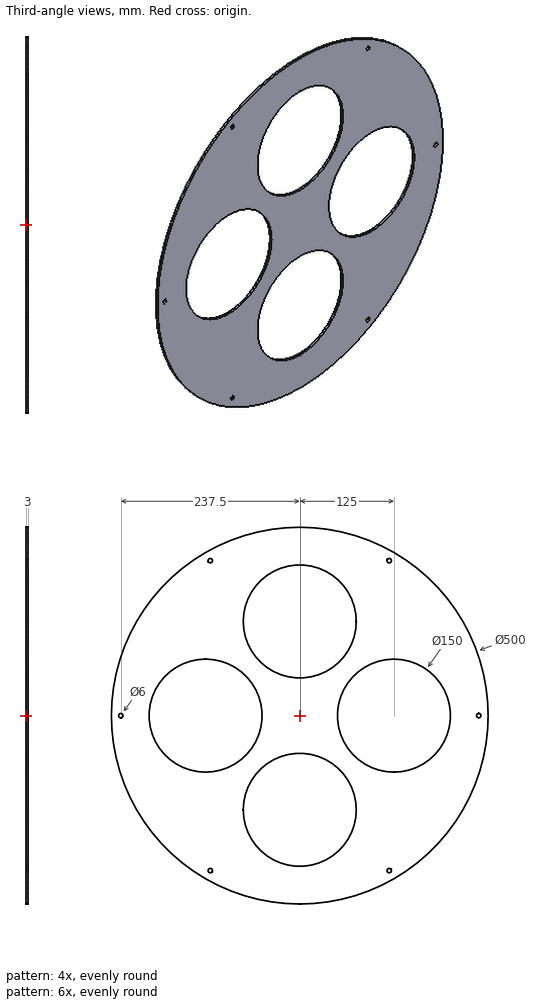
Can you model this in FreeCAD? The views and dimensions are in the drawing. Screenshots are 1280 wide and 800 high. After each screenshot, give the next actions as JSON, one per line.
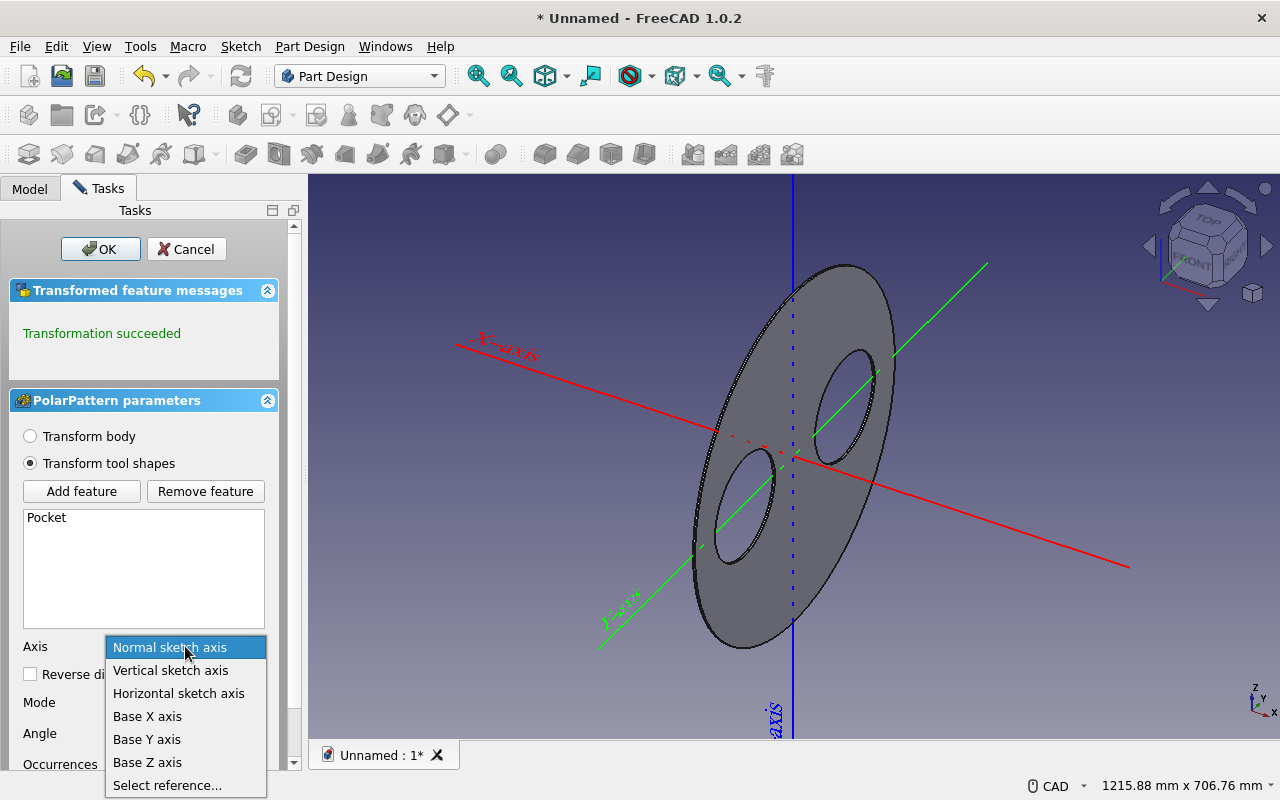
{"action": "left_click", "coordinate": [184, 716]}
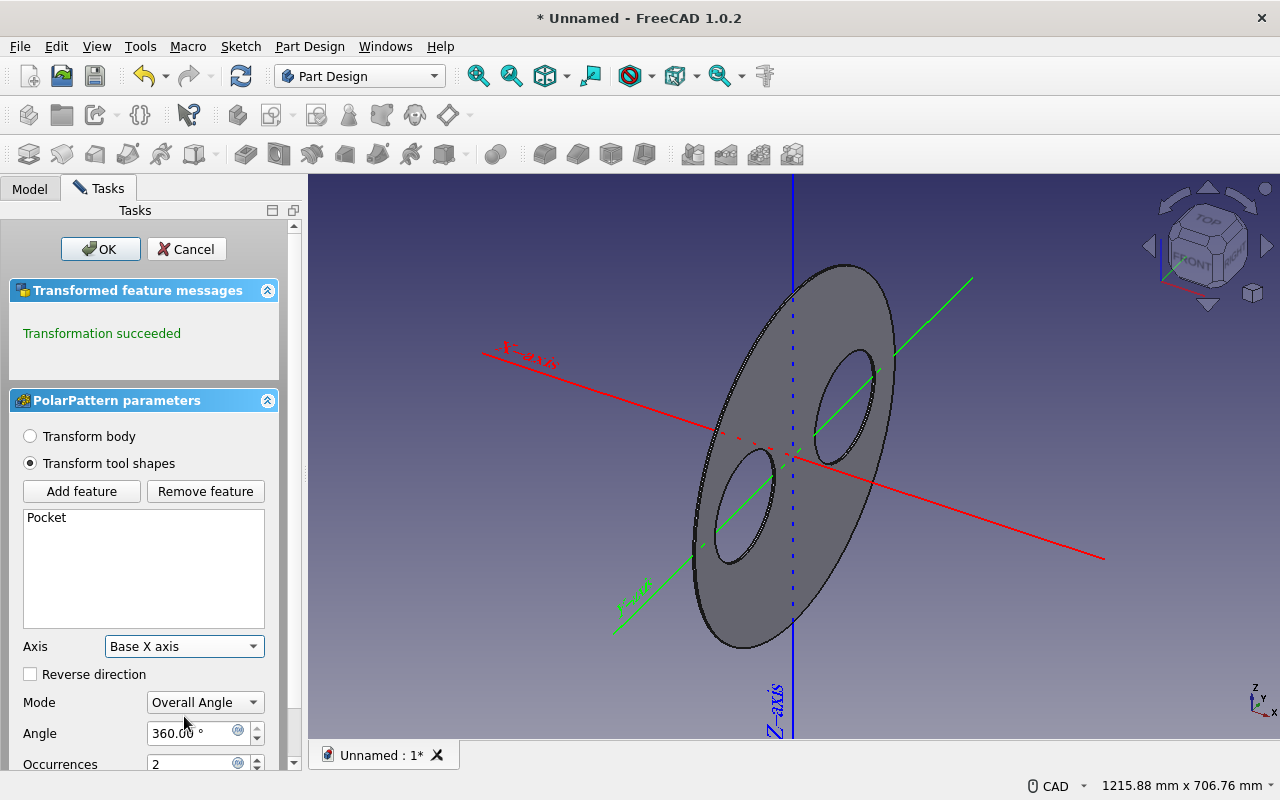
{"action": "scroll", "coordinate": [294, 495], "scroll_direction": "down", "scroll_amount": 2}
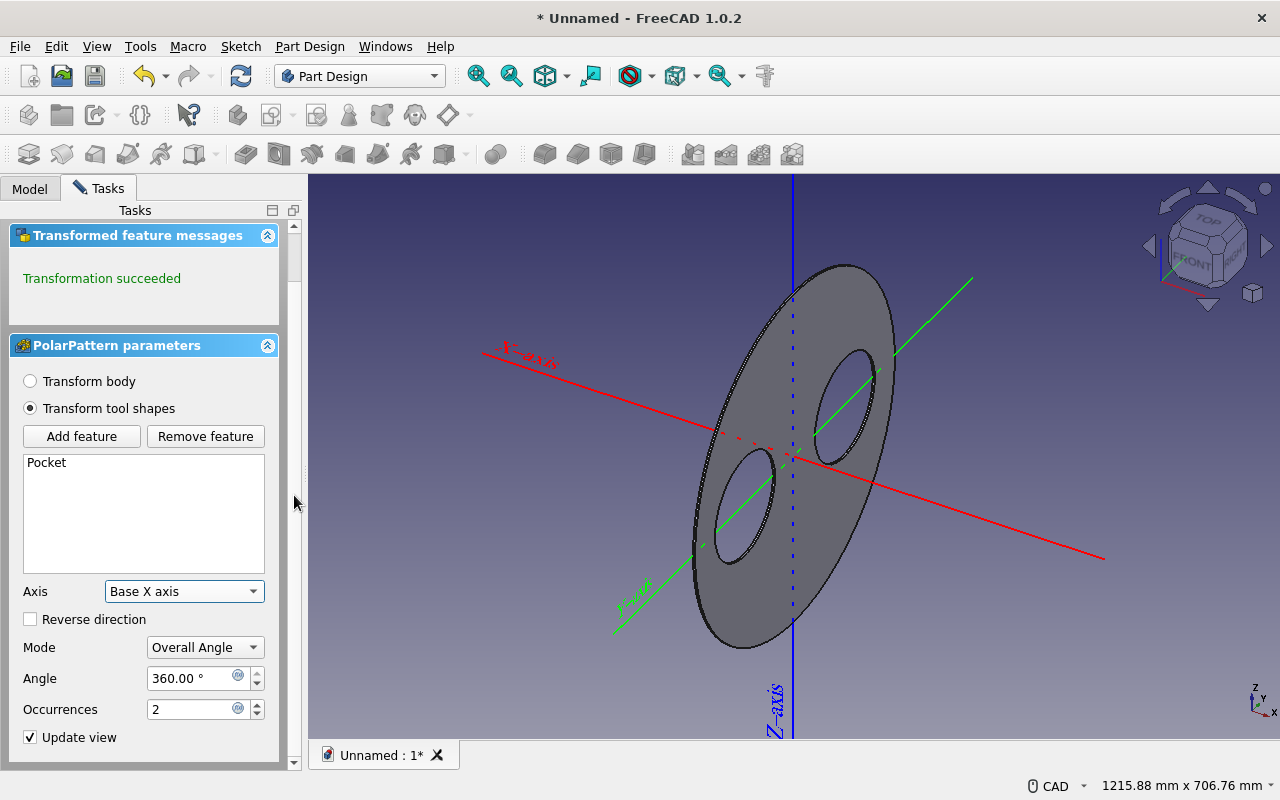
{"action": "triple_click", "coordinate": [199, 710]}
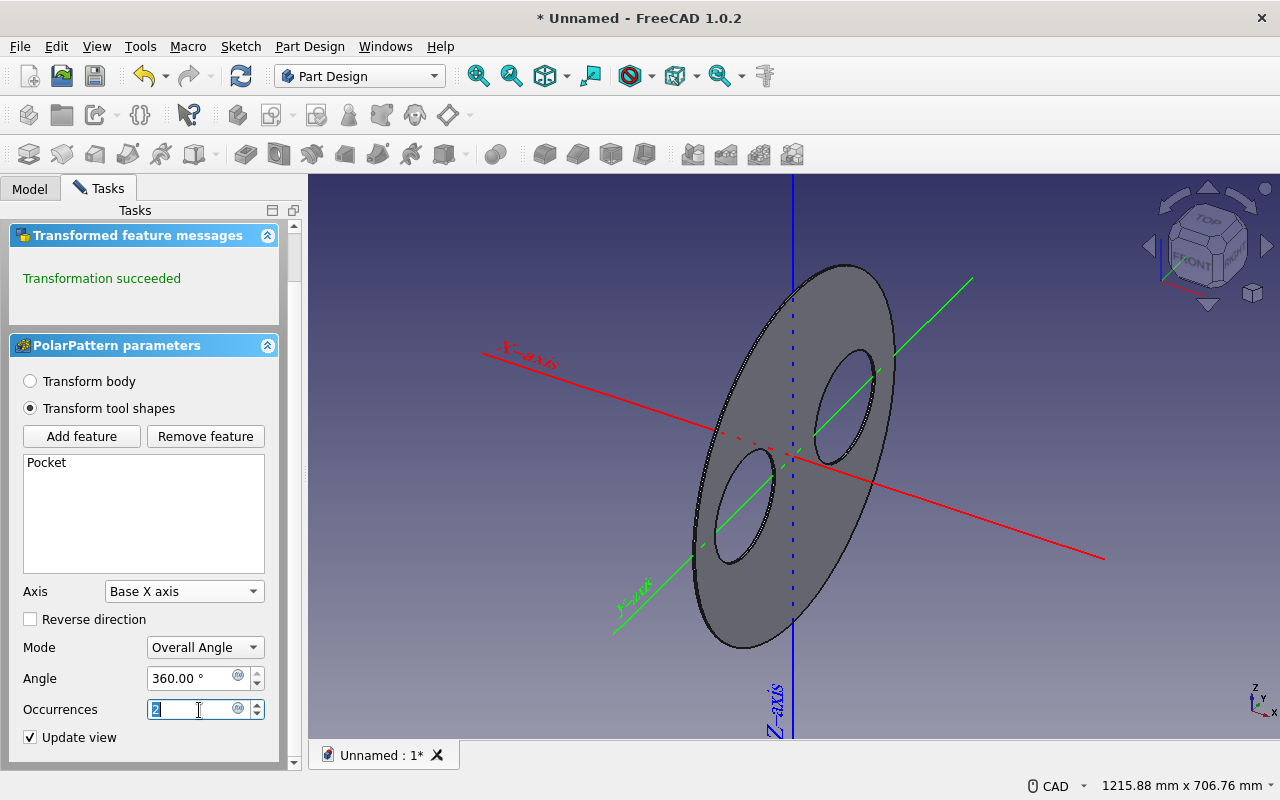
{"action": "type", "text": "4"}
{"action": "key", "text": "Tab"}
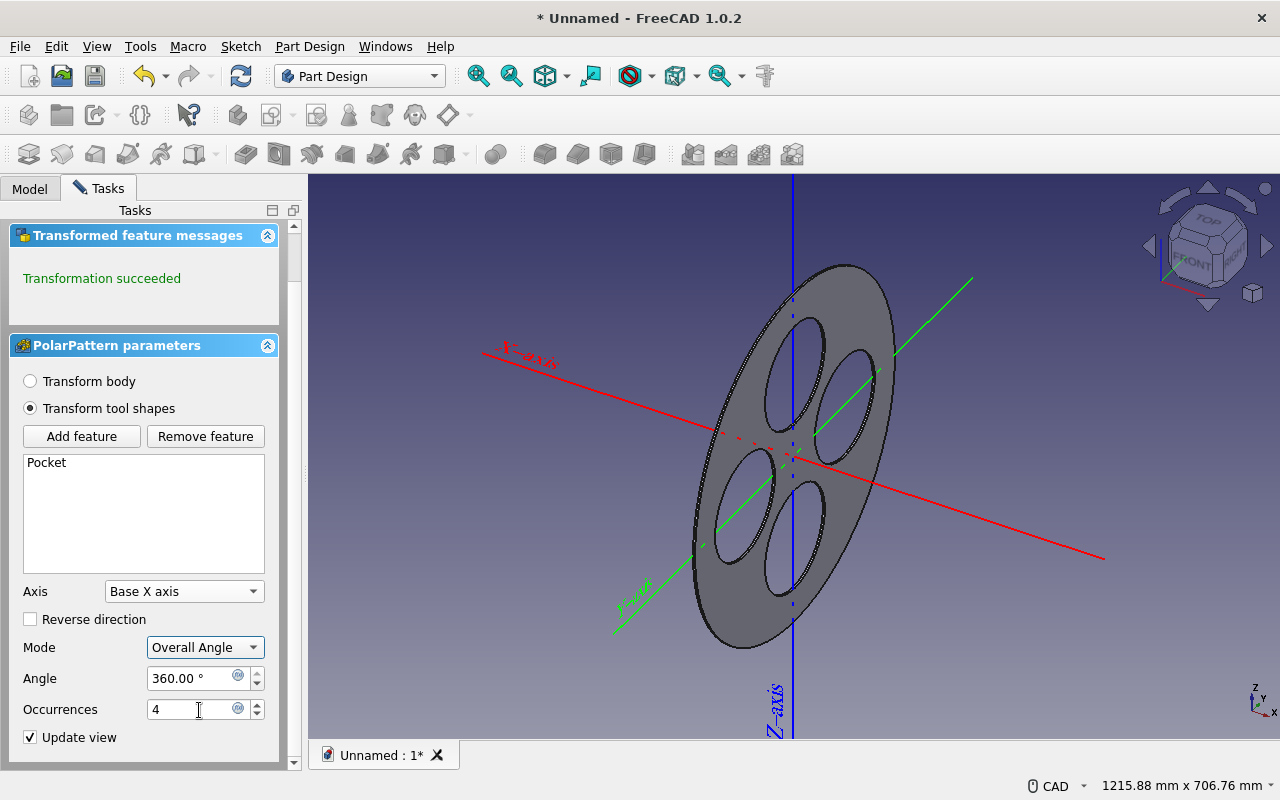
{"action": "scroll", "coordinate": [294, 495], "scroll_direction": "up", "scroll_amount": 2}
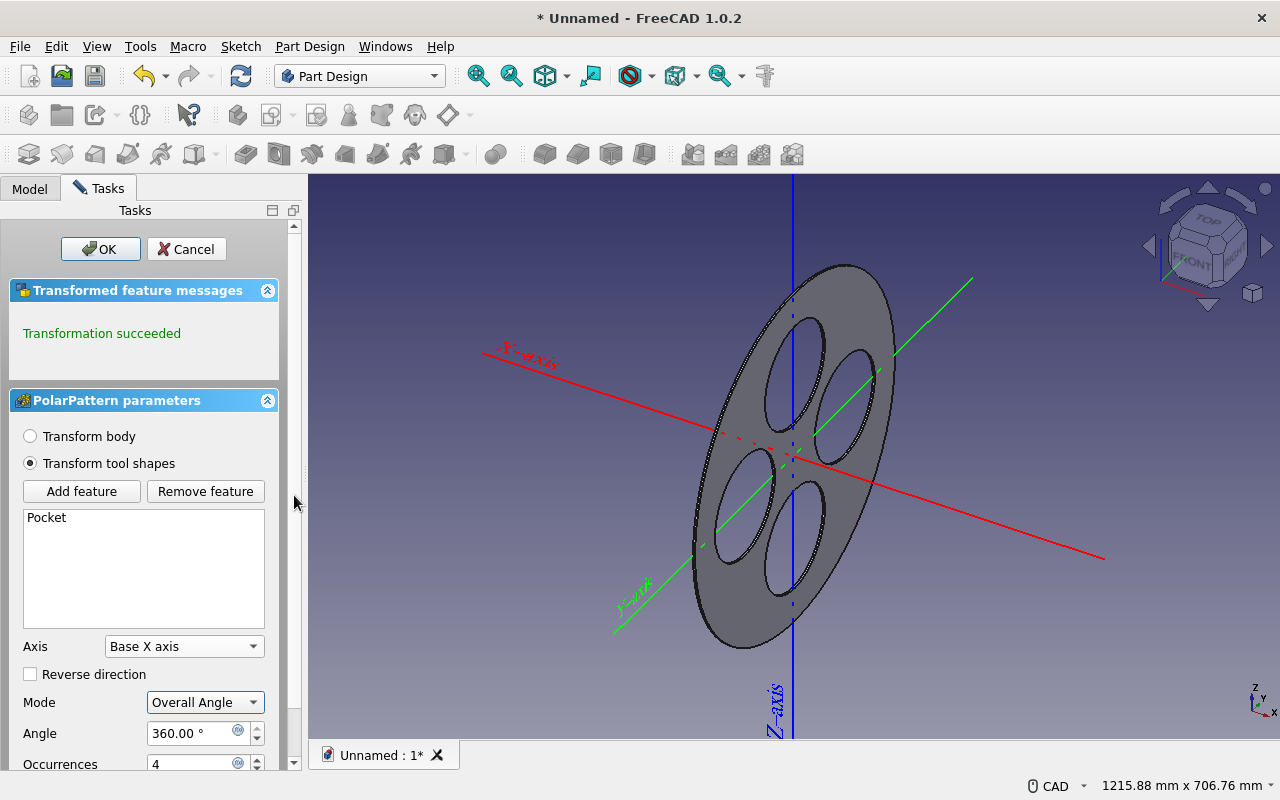
{"action": "left_click", "coordinate": [101, 249]}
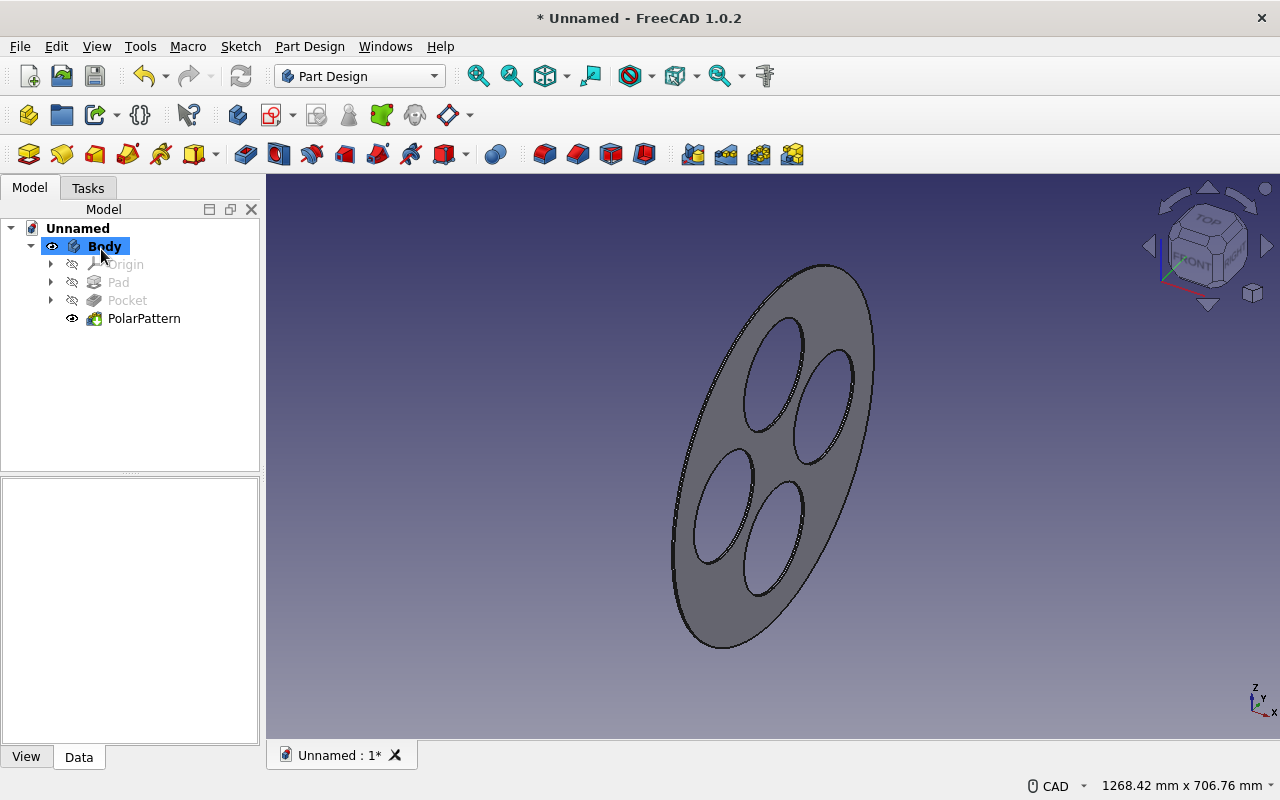
{"action": "left_click", "coordinate": [774, 456]}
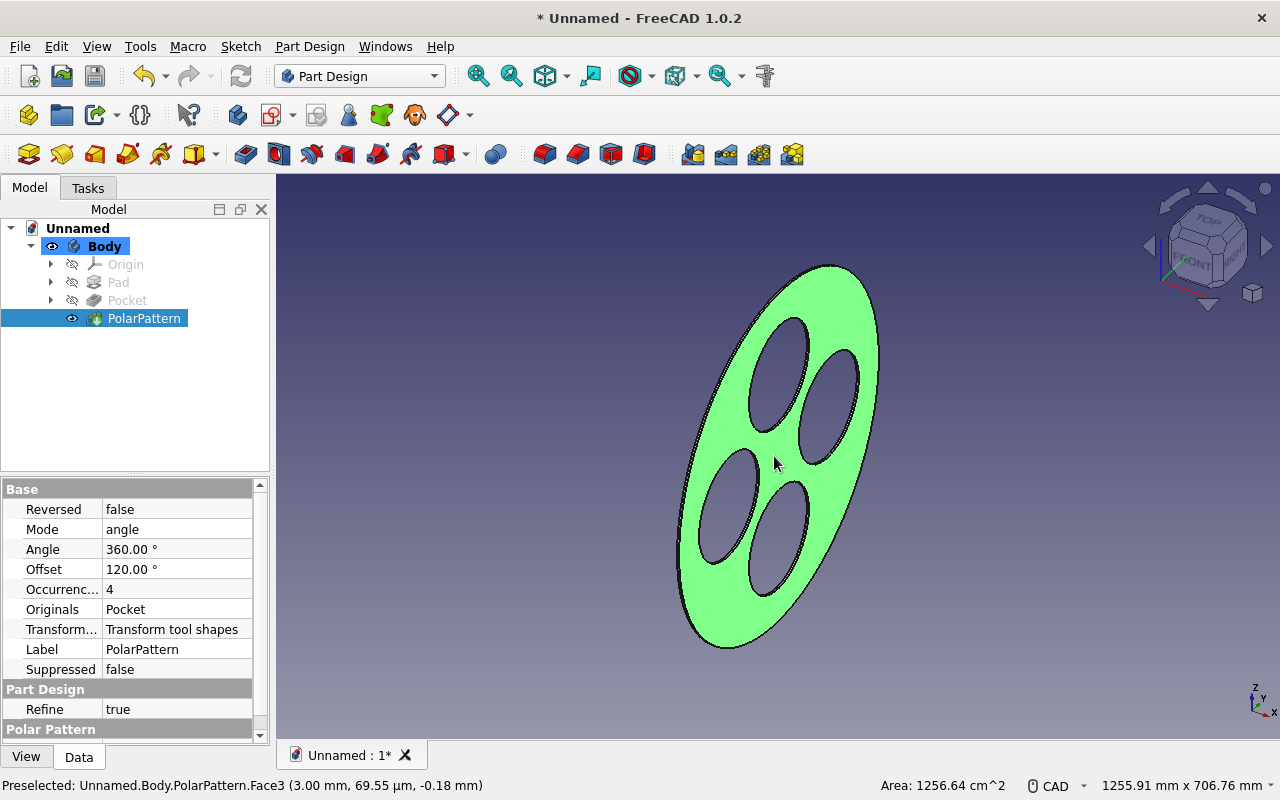
{"action": "left_click", "coordinate": [270, 116]}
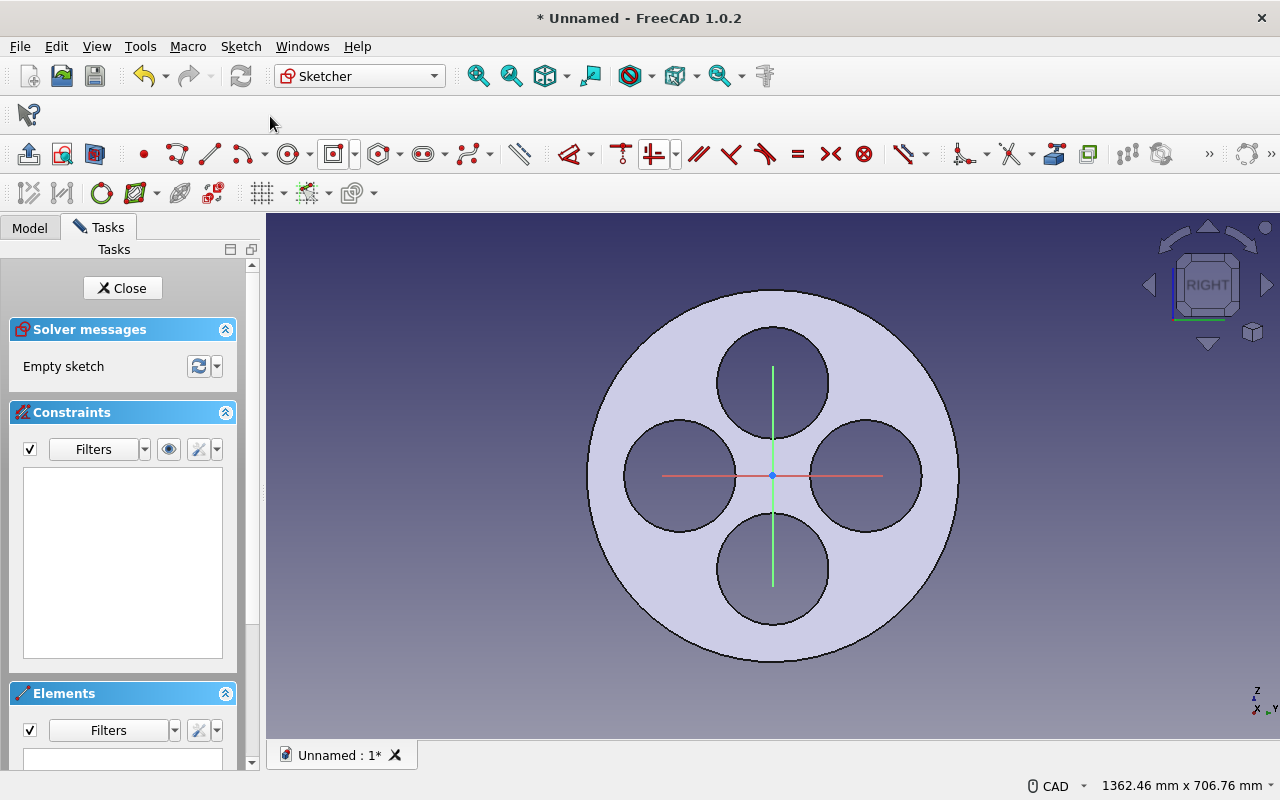
{"action": "scroll", "coordinate": [590, 476], "scroll_direction": "up", "scroll_amount": 15}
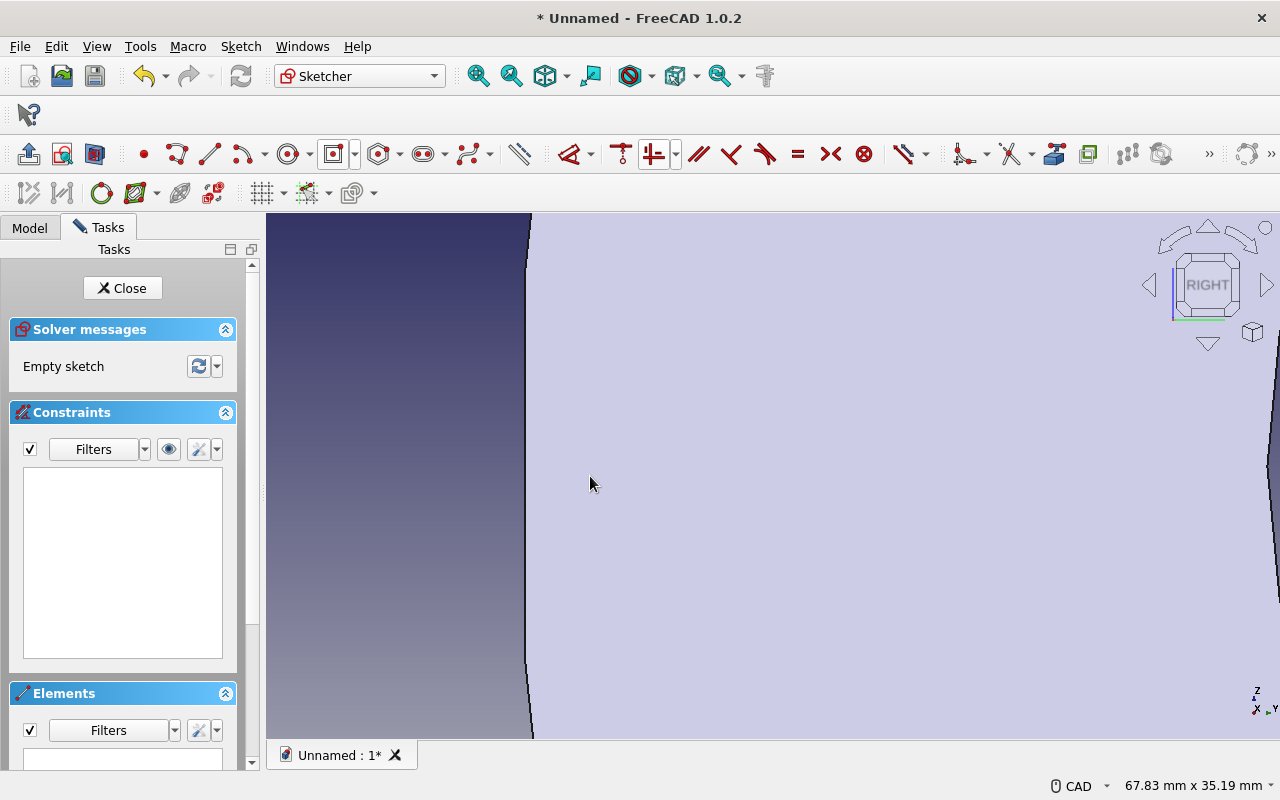
{"action": "scroll", "coordinate": [708, 463], "scroll_direction": "up", "scroll_amount": 7}